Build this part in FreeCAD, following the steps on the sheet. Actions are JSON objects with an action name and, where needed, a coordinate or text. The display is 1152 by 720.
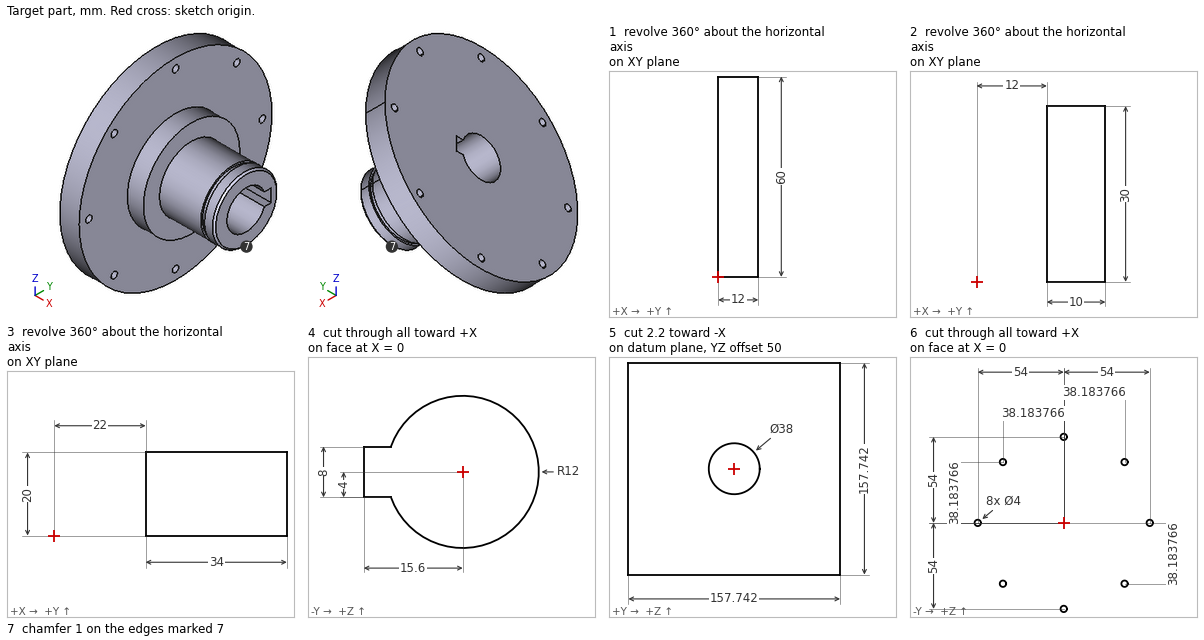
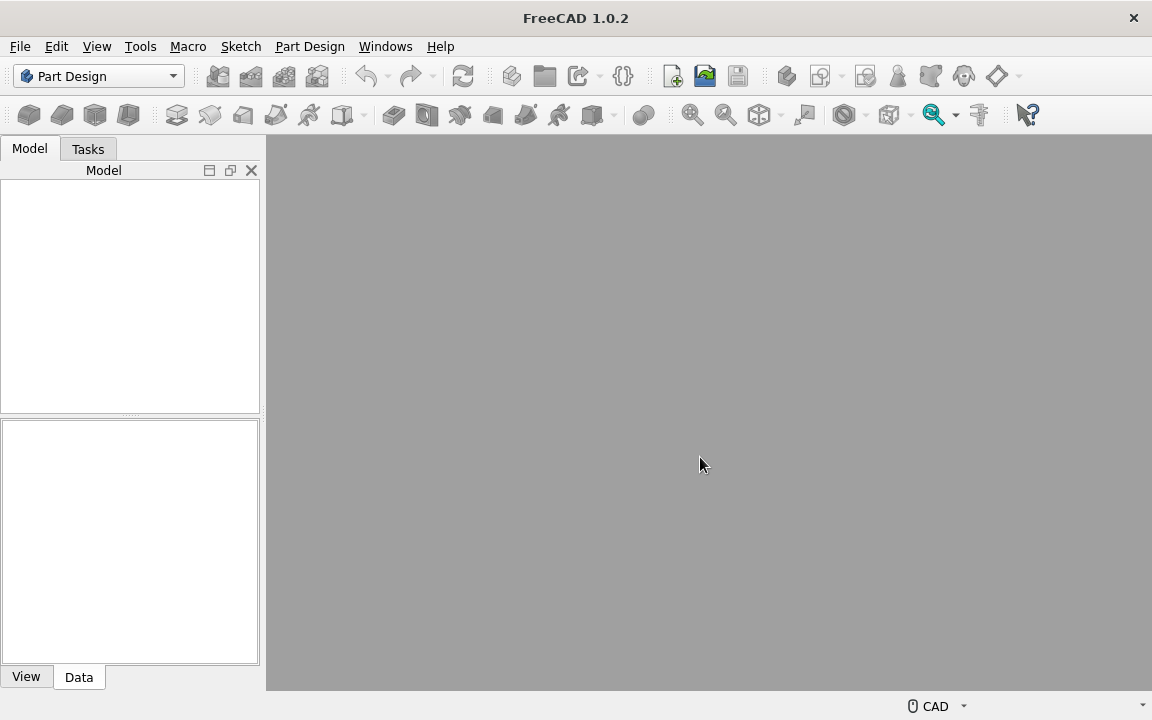
{"action": "left_click", "coordinate": [672, 76]}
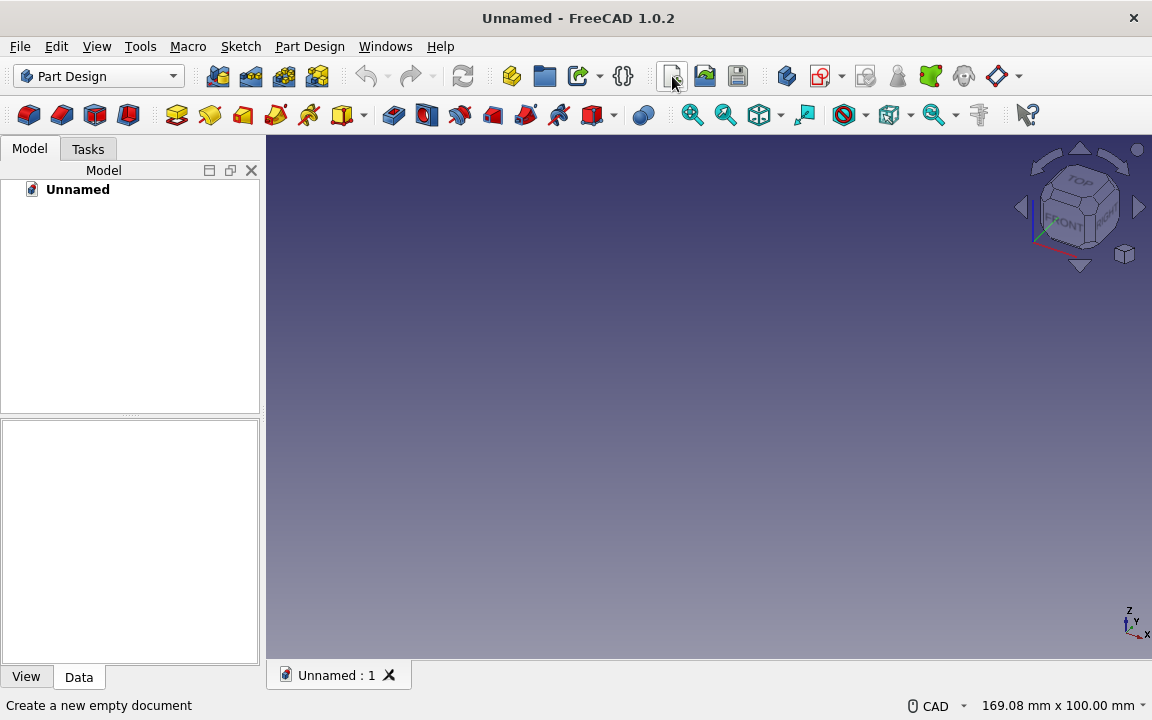
{"action": "left_click", "coordinate": [820, 76]}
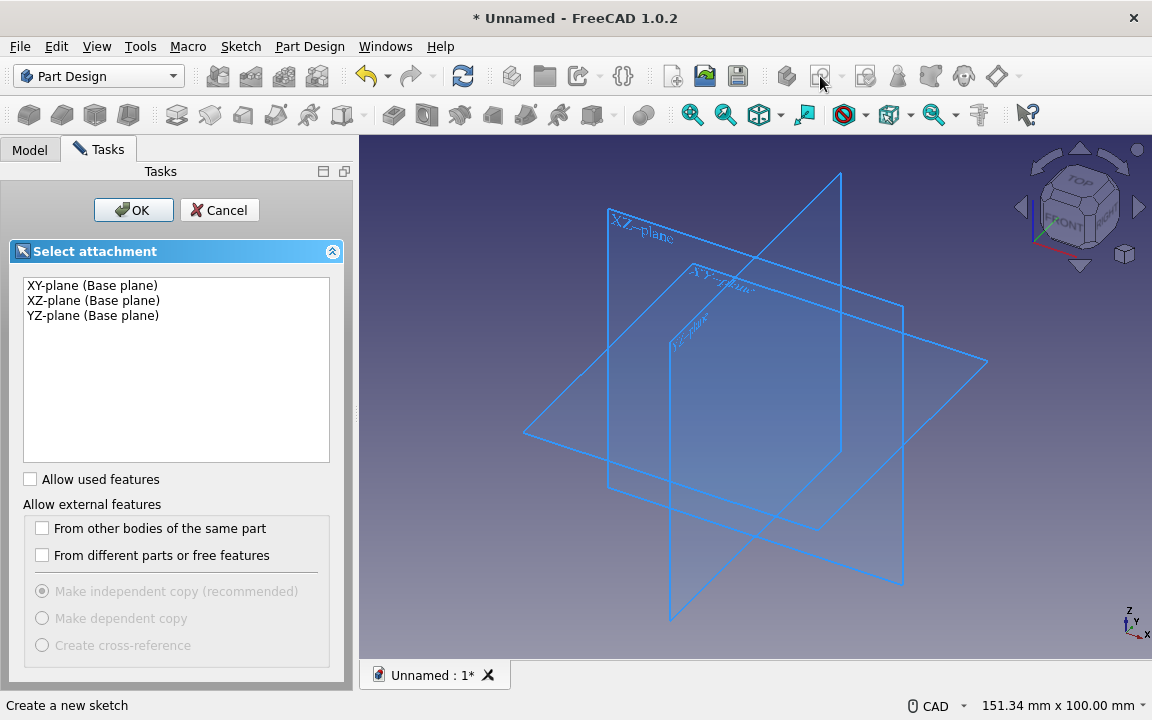
{"action": "left_click", "coordinate": [84, 286]}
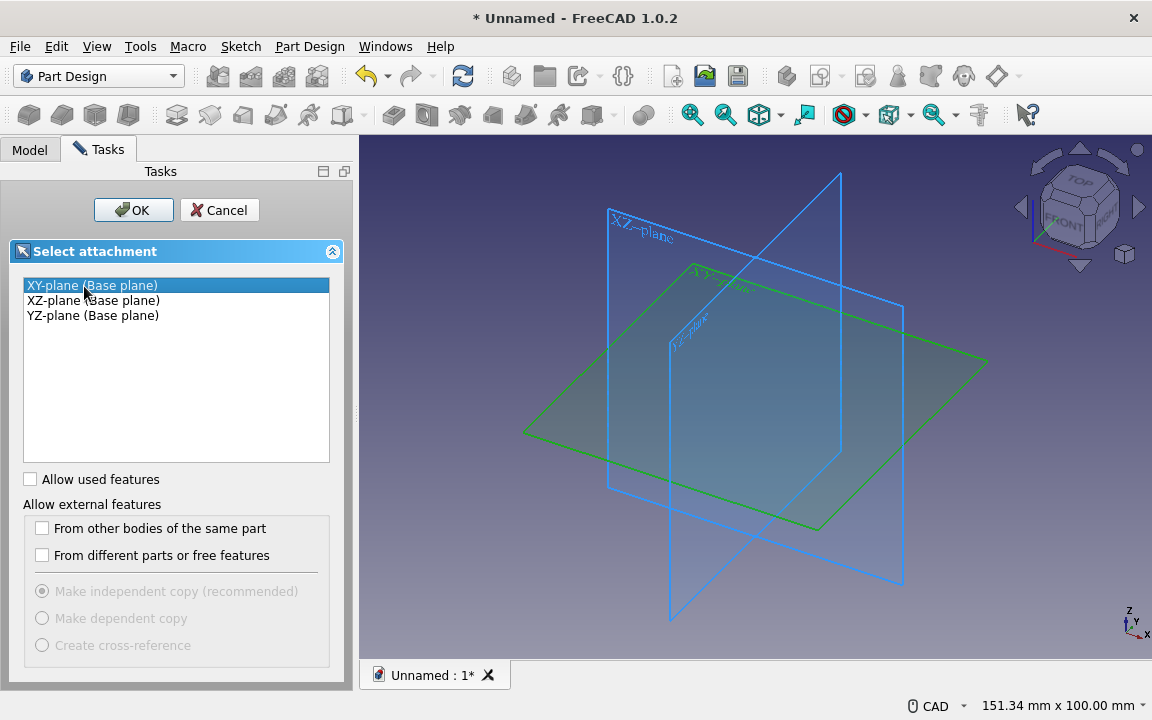
{"action": "left_click", "coordinate": [134, 210]}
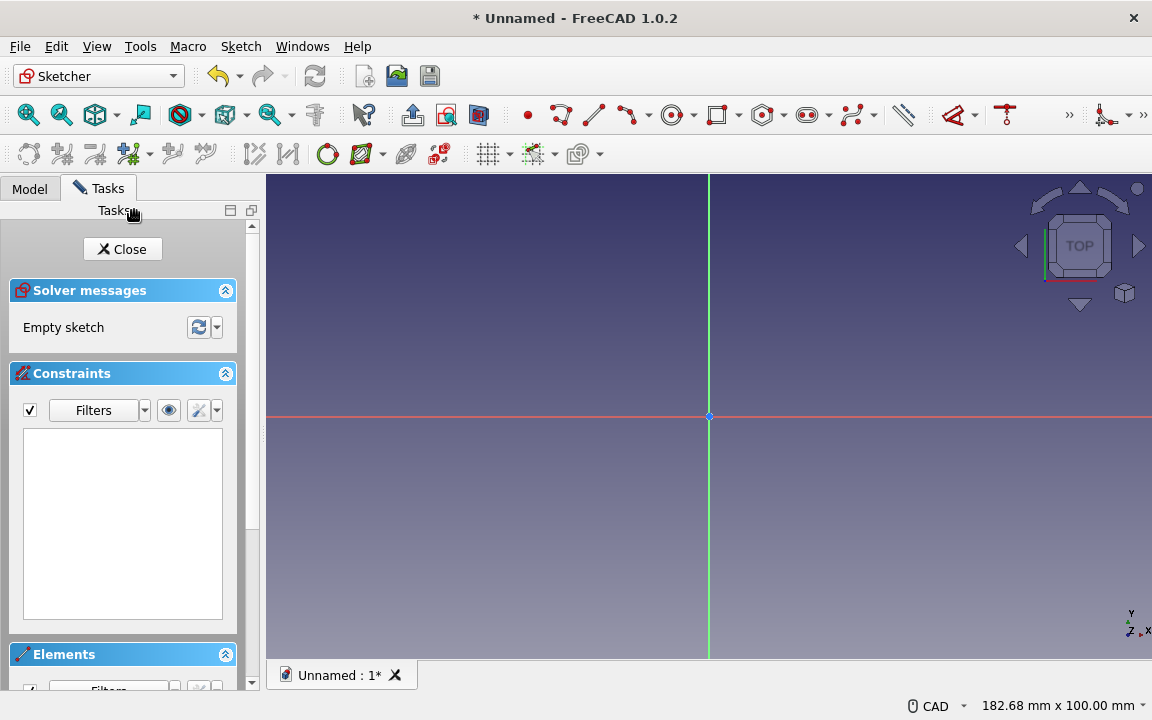
{"action": "scroll", "coordinate": [442, 631], "scroll_direction": "down", "scroll_amount": 2}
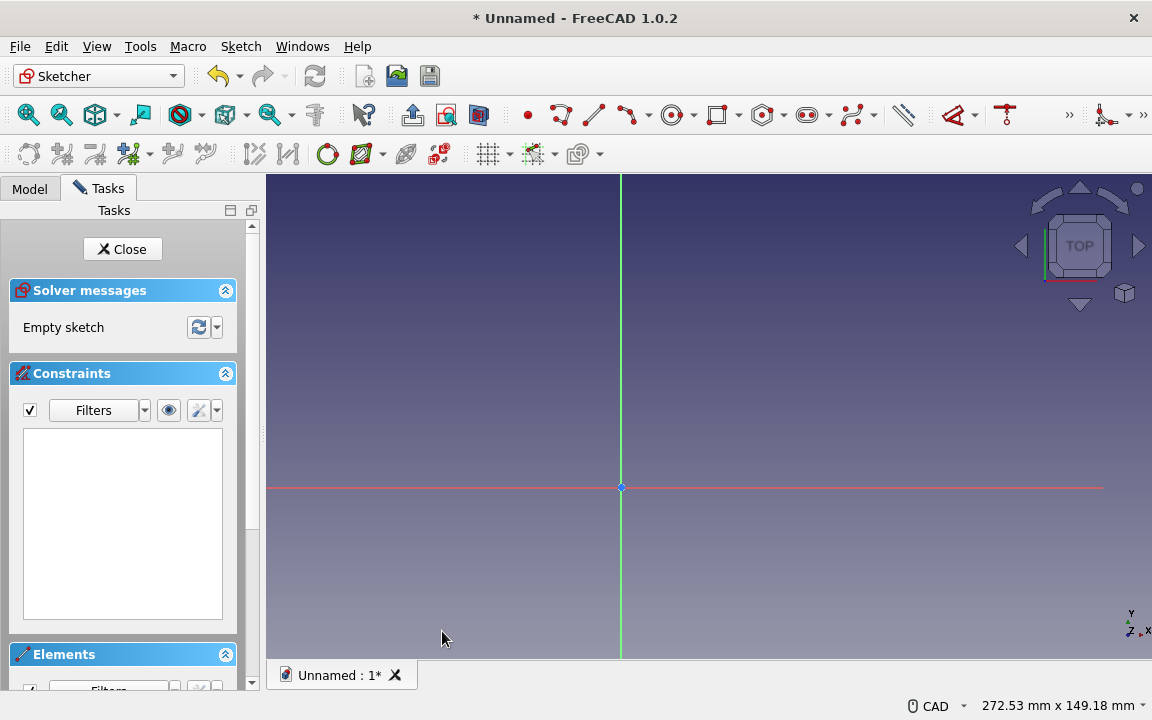
{"action": "scroll", "coordinate": [641, 336], "scroll_direction": "up", "scroll_amount": 2}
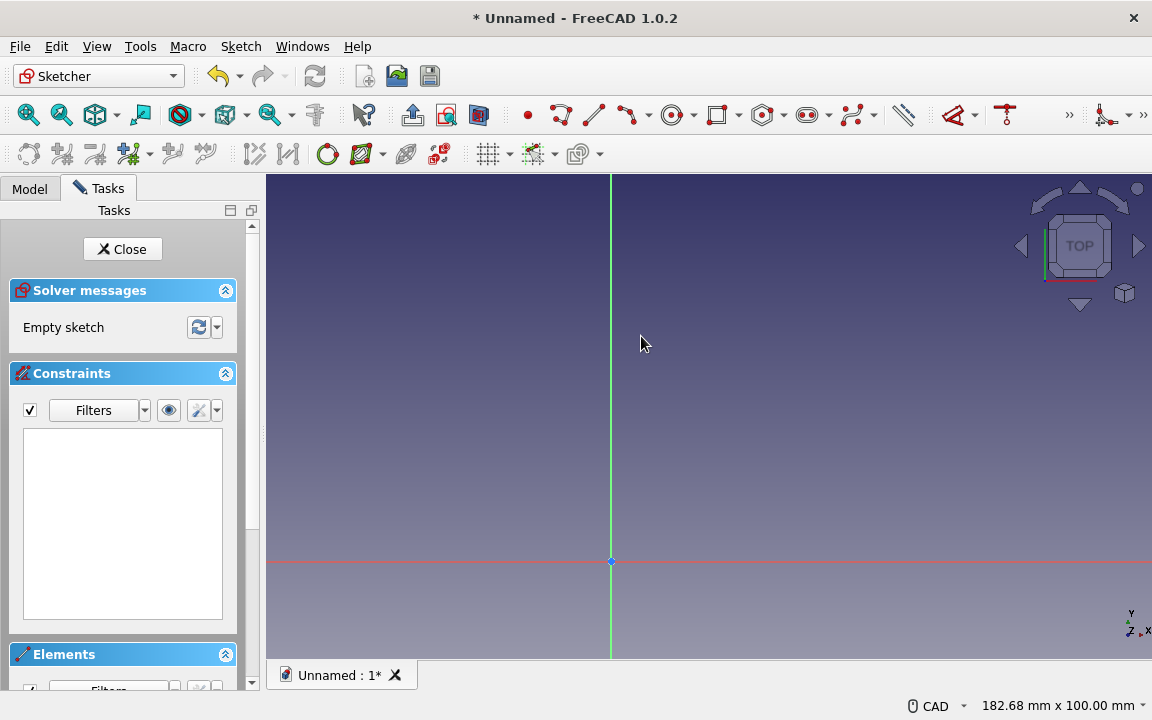
{"action": "left_click", "coordinate": [716, 116]}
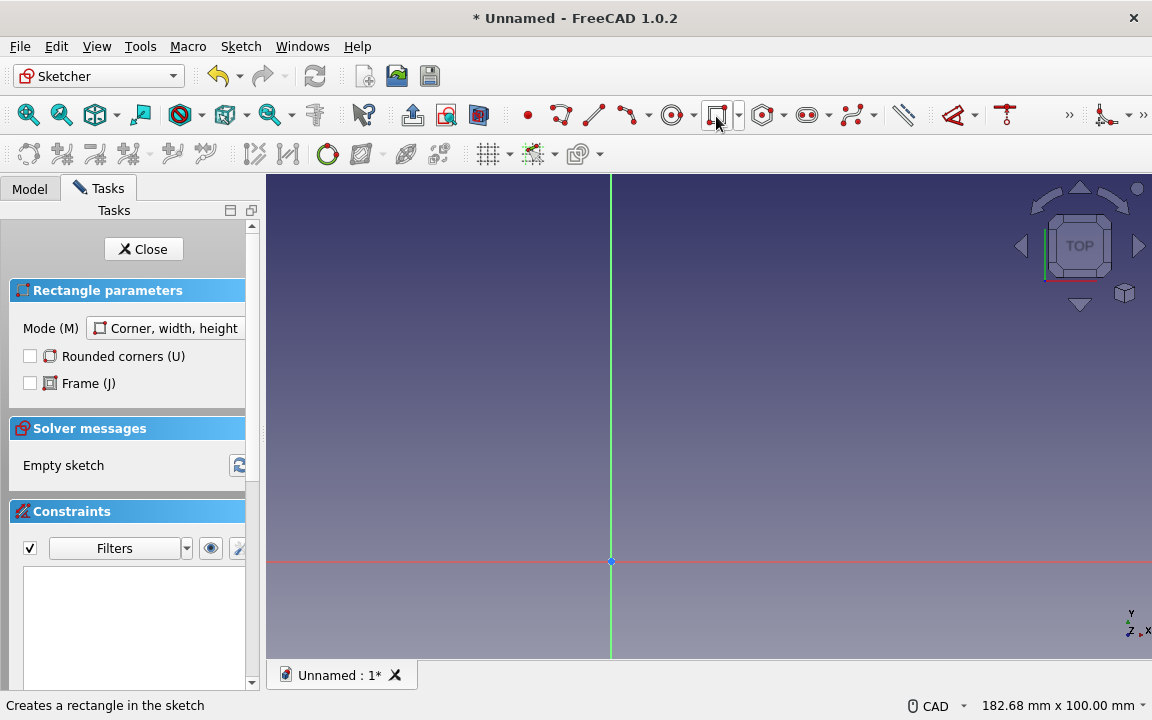
{"action": "left_click", "coordinate": [611, 562]}
{"action": "left_click", "coordinate": [669, 271]}
{"action": "key", "text": "Escape"}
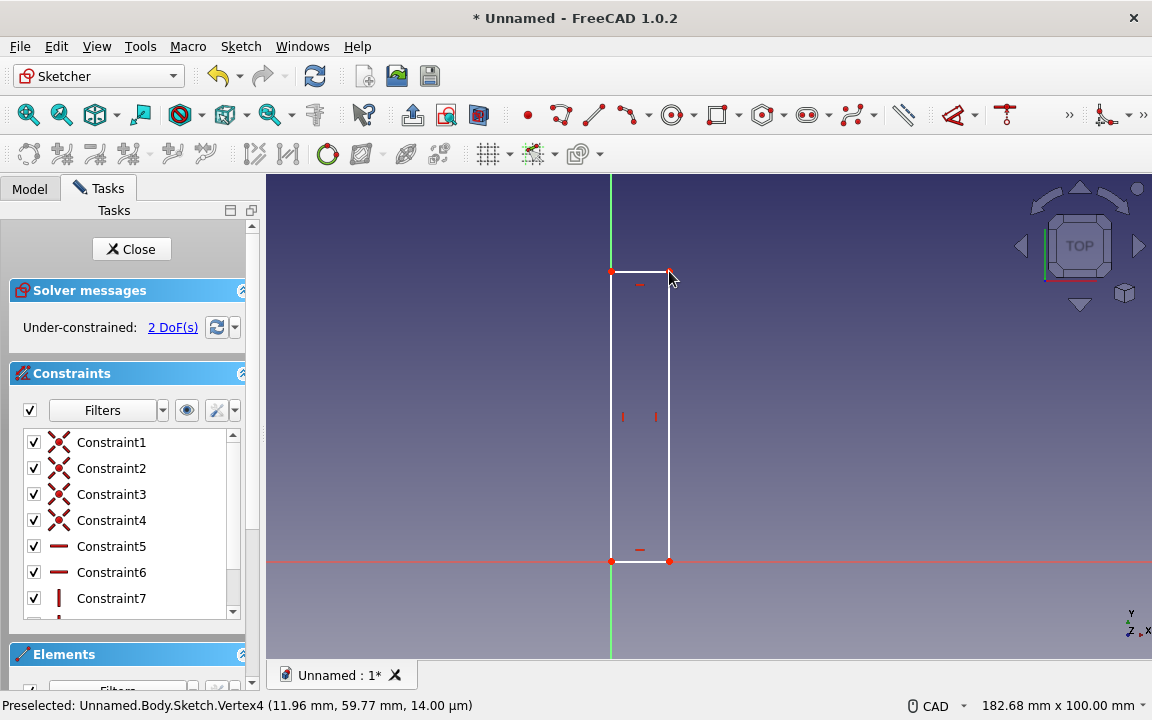
{"action": "left_click", "coordinate": [952, 116]}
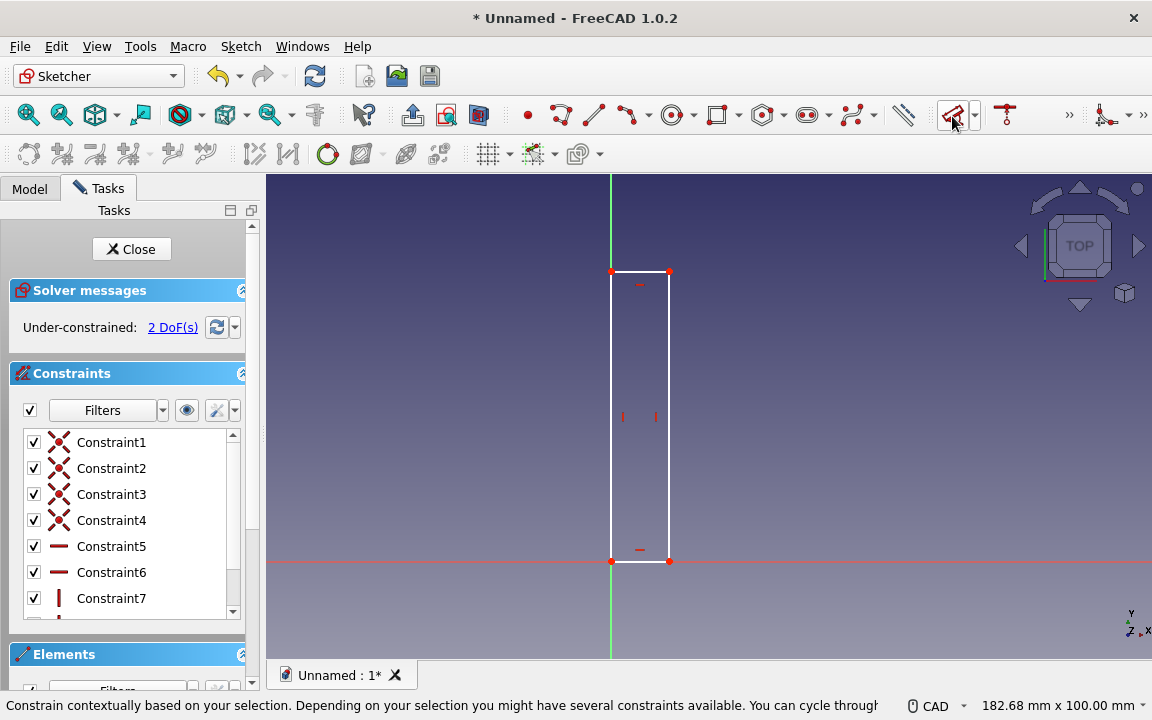
{"action": "left_click", "coordinate": [628, 562]}
{"action": "left_click", "coordinate": [640, 596]}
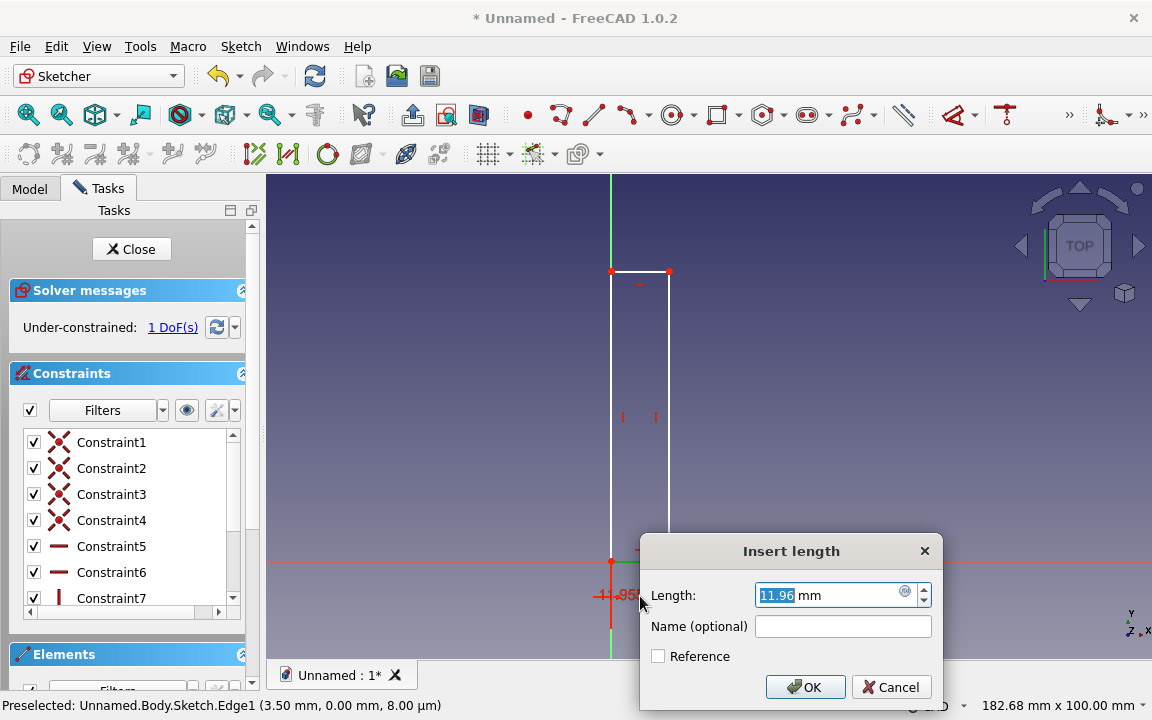
{"action": "type", "text": "12"}
{"action": "key", "text": "Return"}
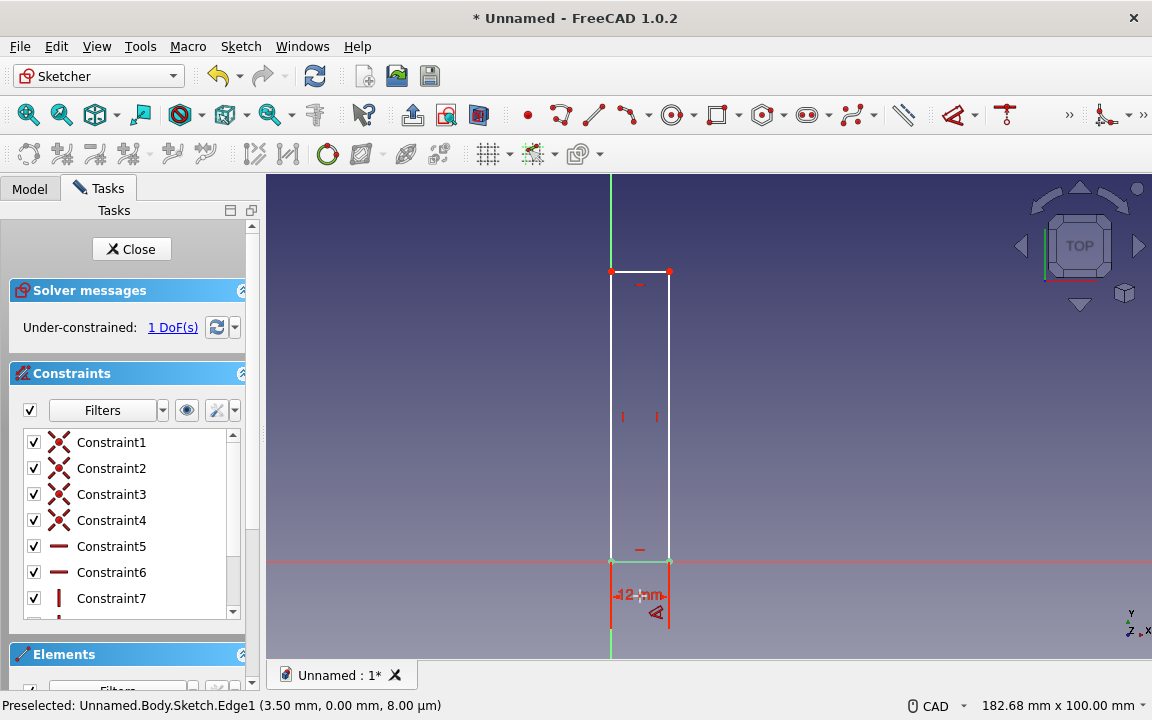
{"action": "left_click", "coordinate": [669, 475]}
{"action": "left_click", "coordinate": [703, 417]}